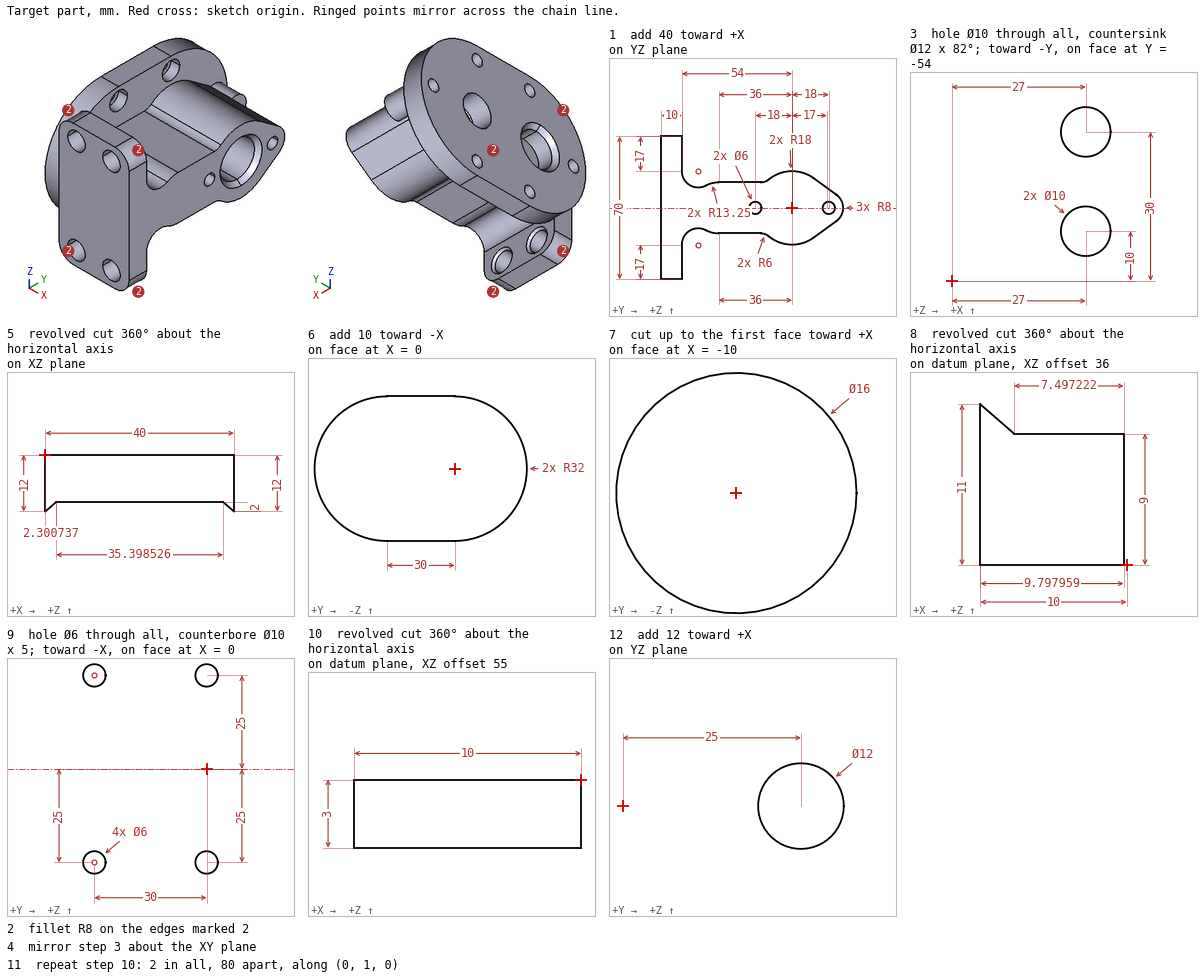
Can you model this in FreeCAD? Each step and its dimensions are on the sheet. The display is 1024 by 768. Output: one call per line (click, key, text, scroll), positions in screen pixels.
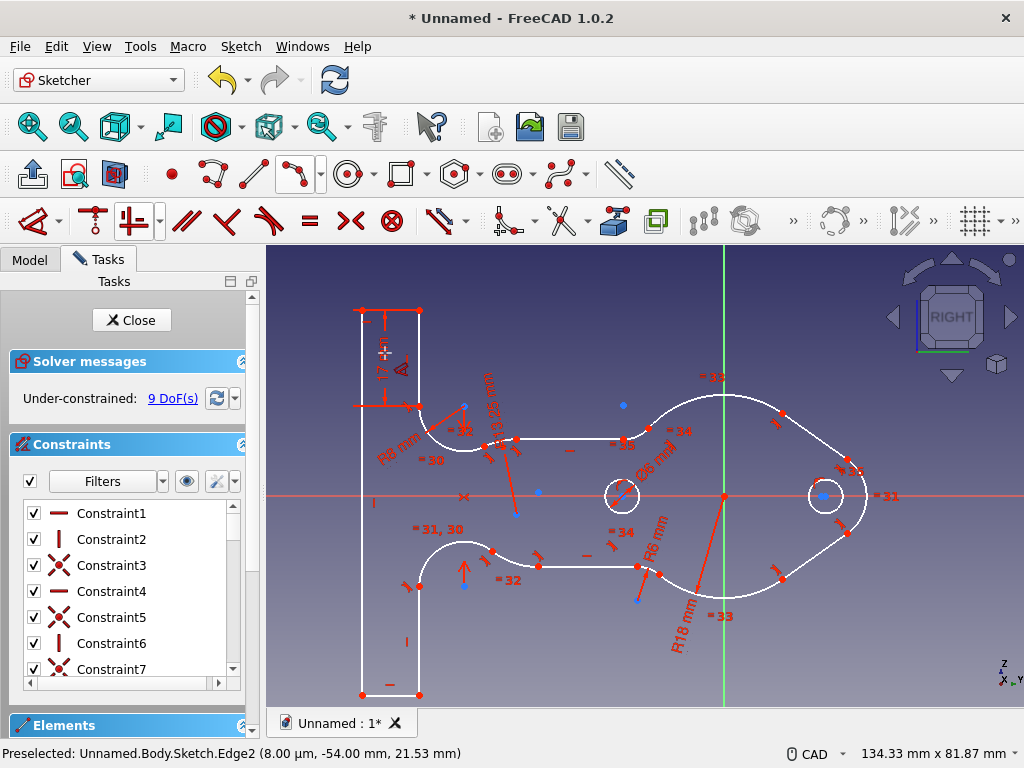
click(402, 310)
click(391, 276)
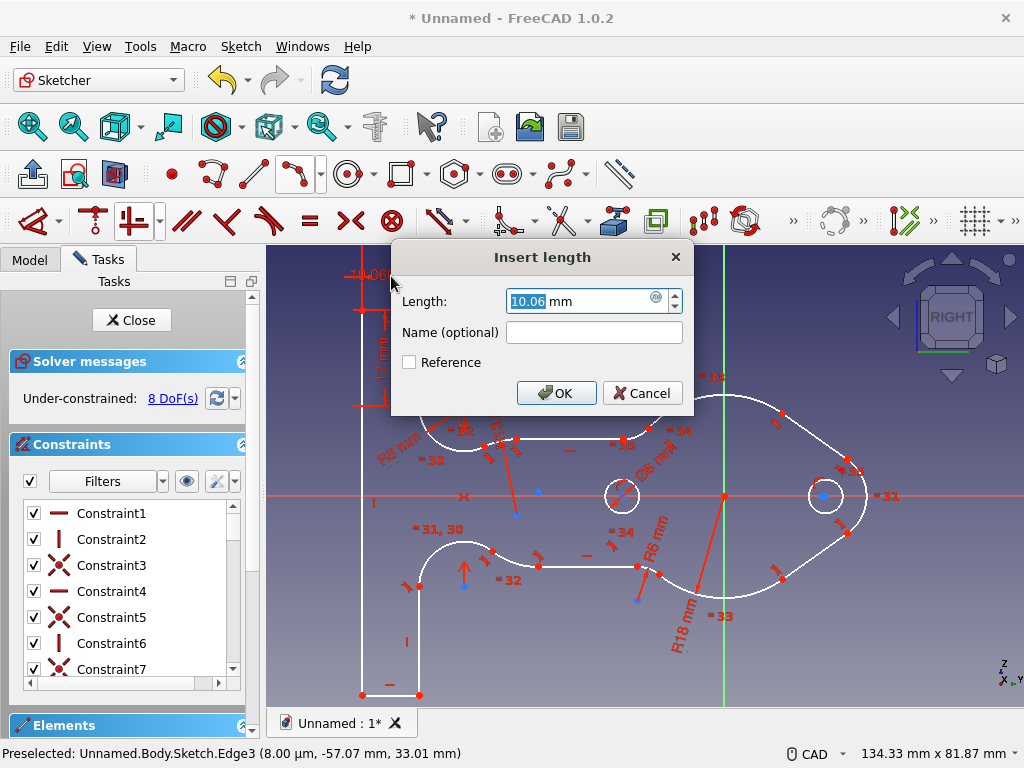
text(10)
key(Return)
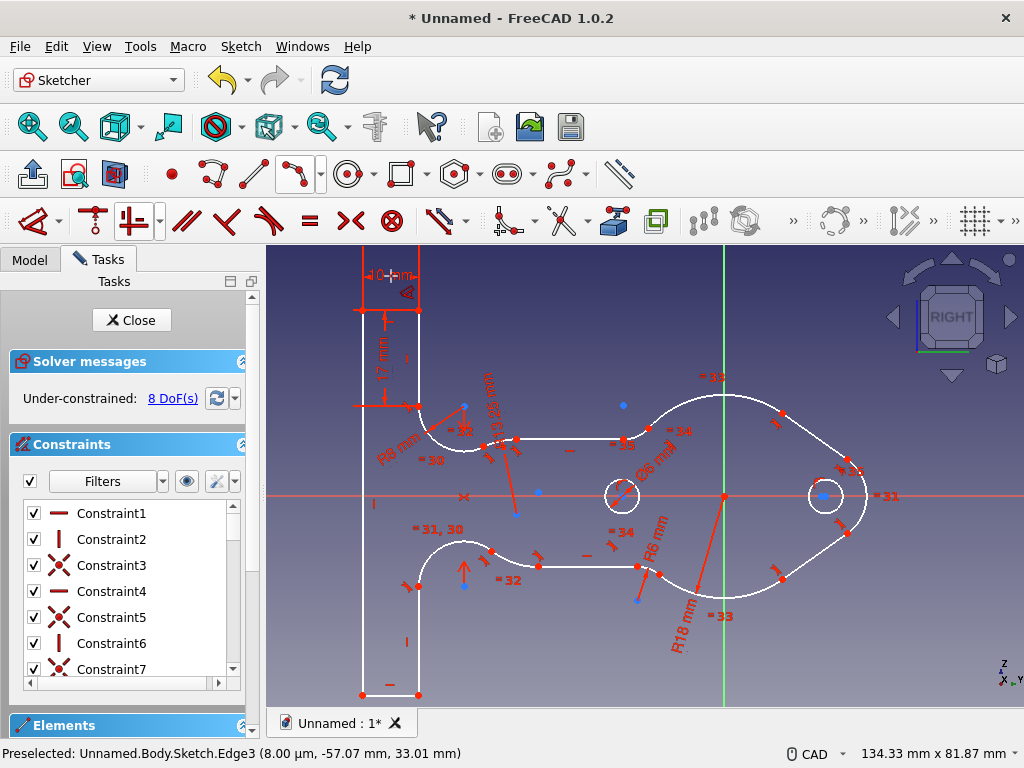
click(363, 426)
click(329, 410)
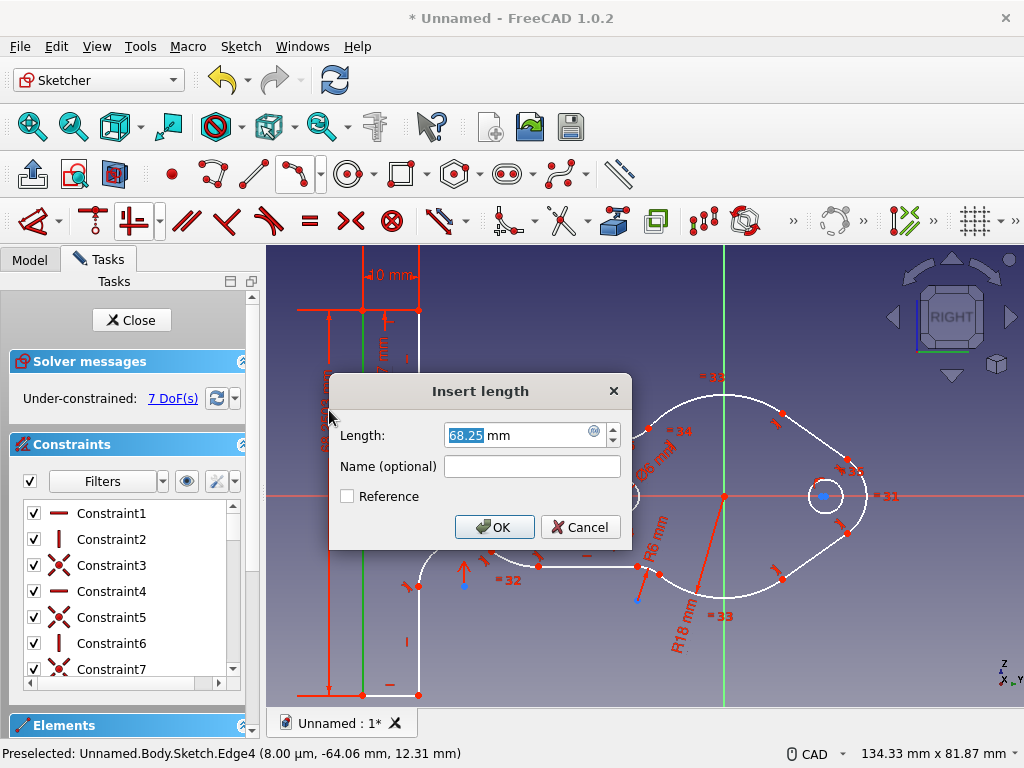
text(70)
key(Return)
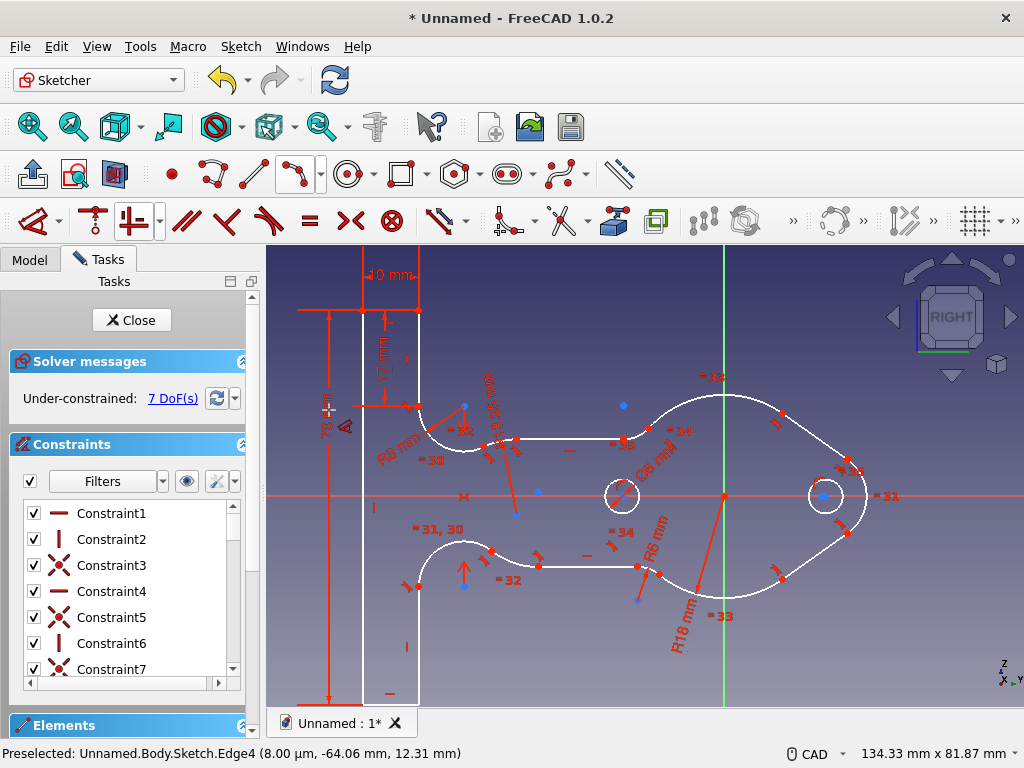
click(419, 670)
click(385, 633)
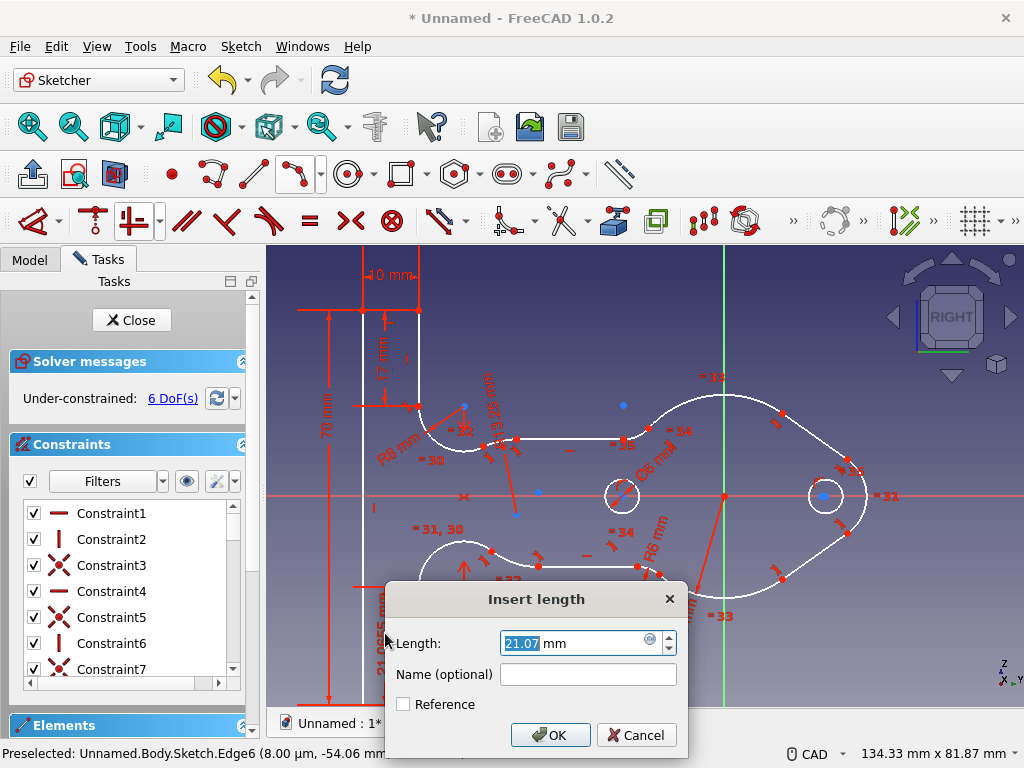
text(17)
key(Return)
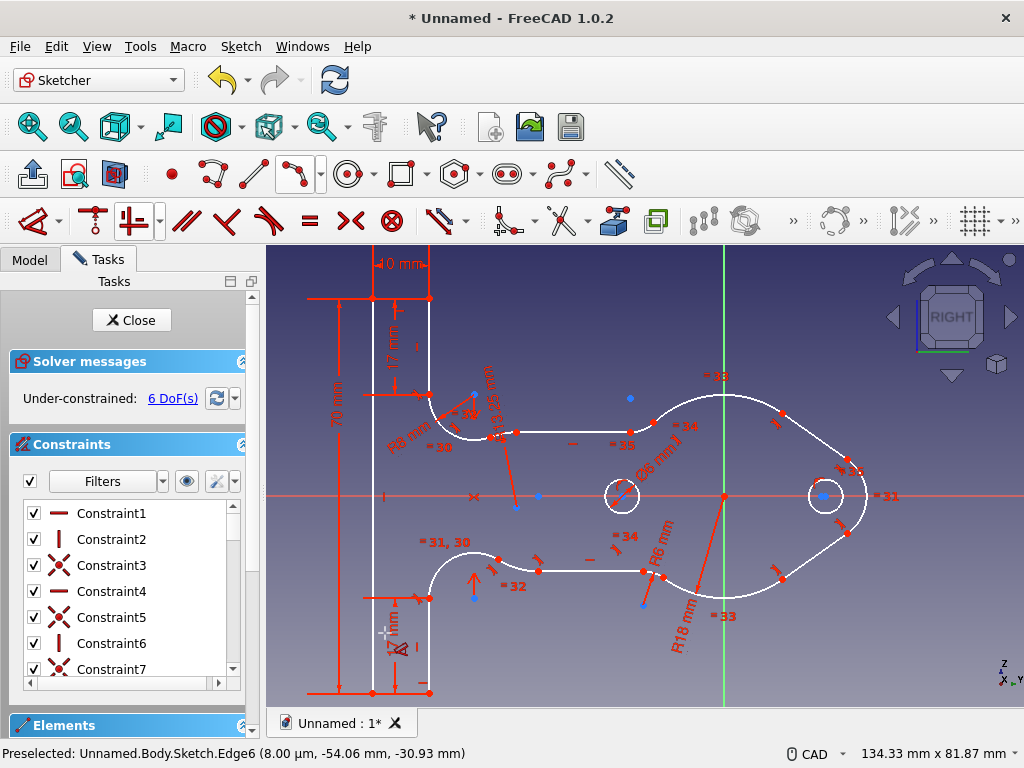
click(622, 496)
click(673, 438)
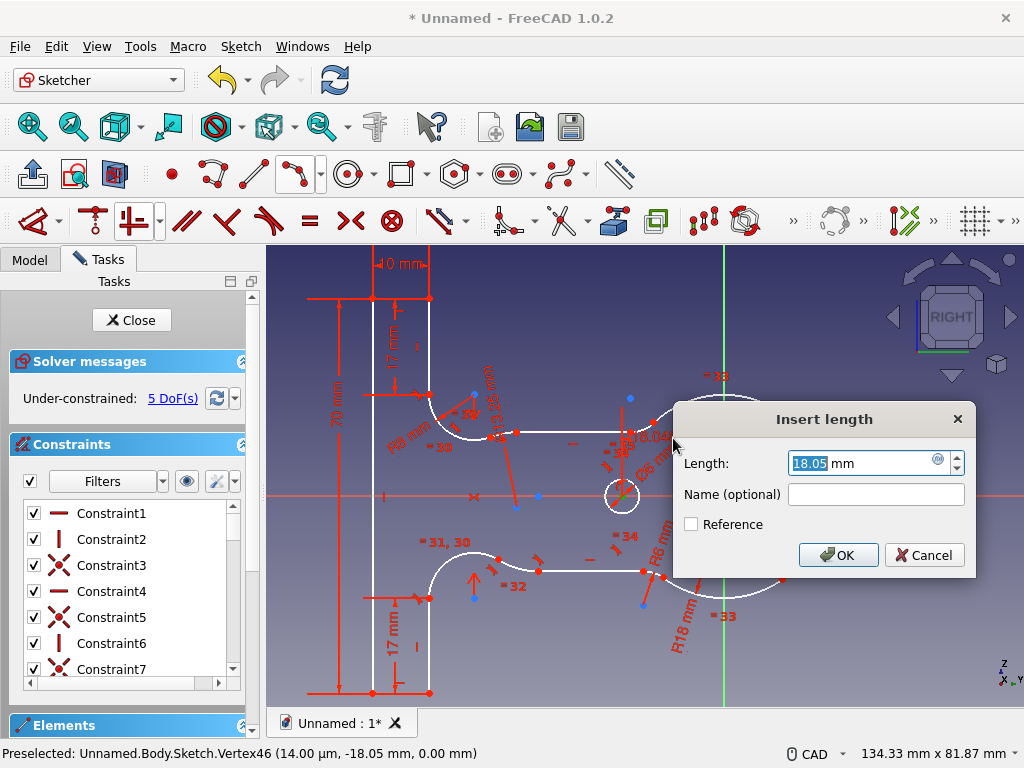
text(18)
key(Return)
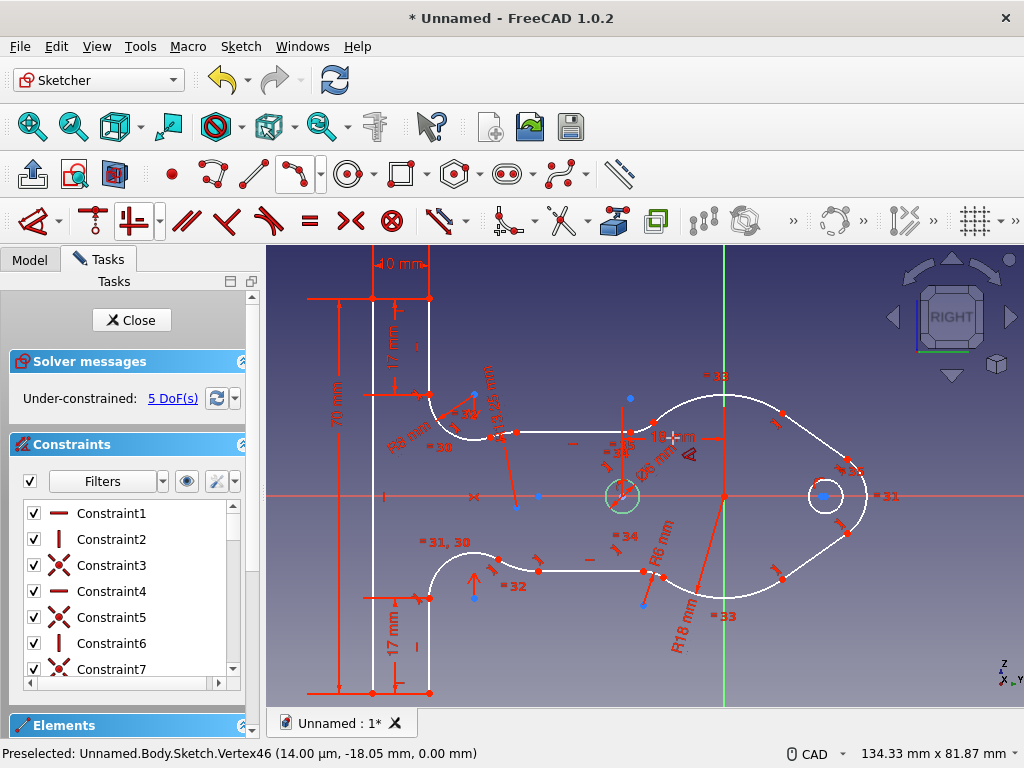
scroll(826, 496, up, 6)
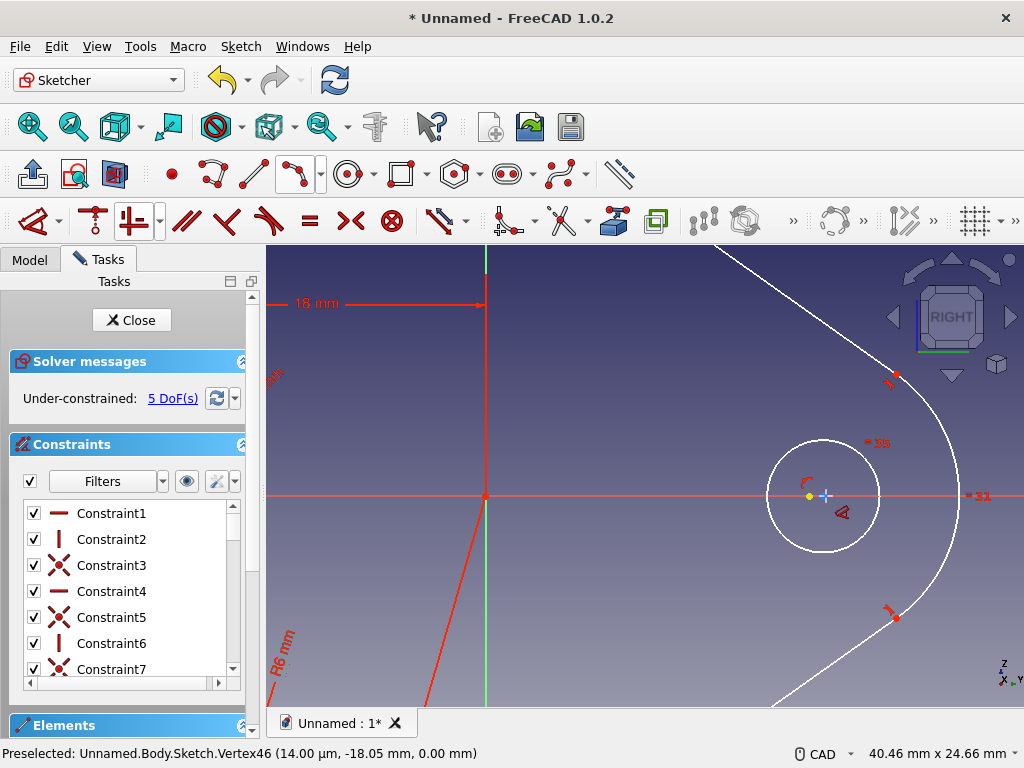
click(823, 496)
click(655, 530)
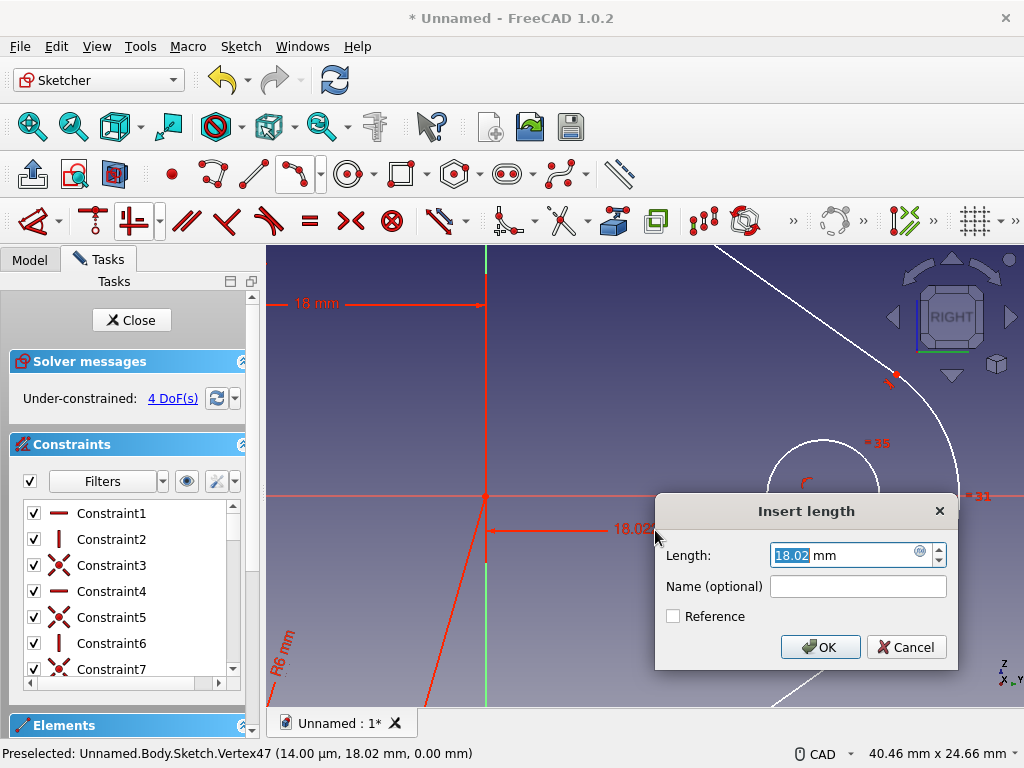
text(18)
key(Return)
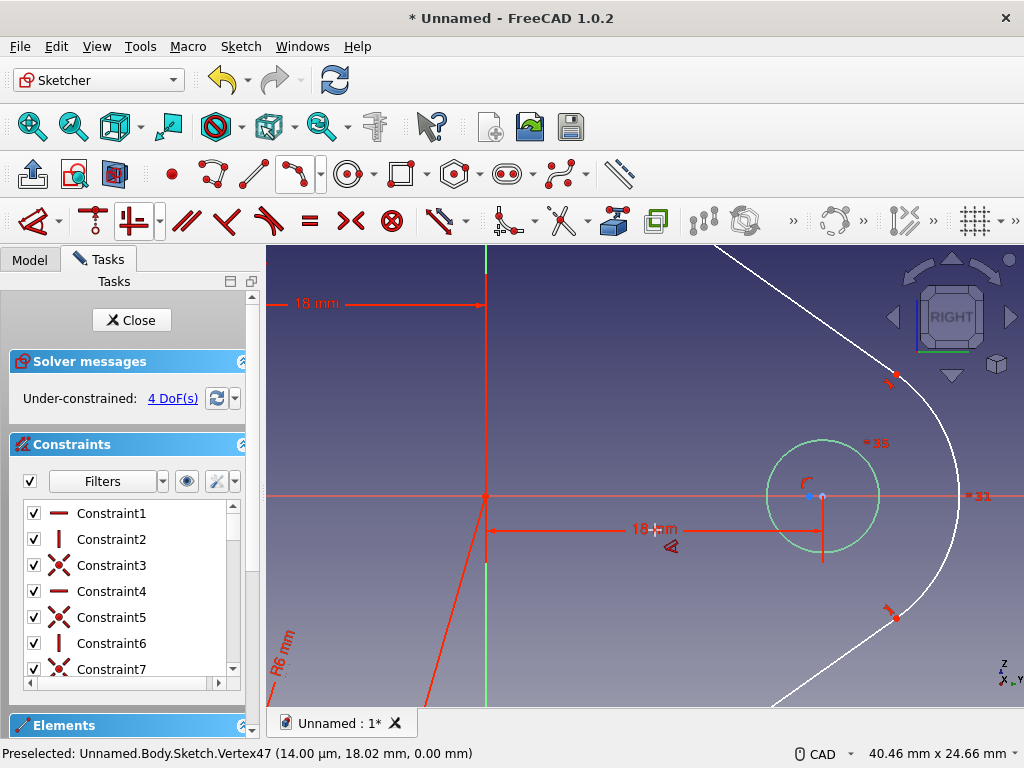
scroll(692, 471, down, 8)